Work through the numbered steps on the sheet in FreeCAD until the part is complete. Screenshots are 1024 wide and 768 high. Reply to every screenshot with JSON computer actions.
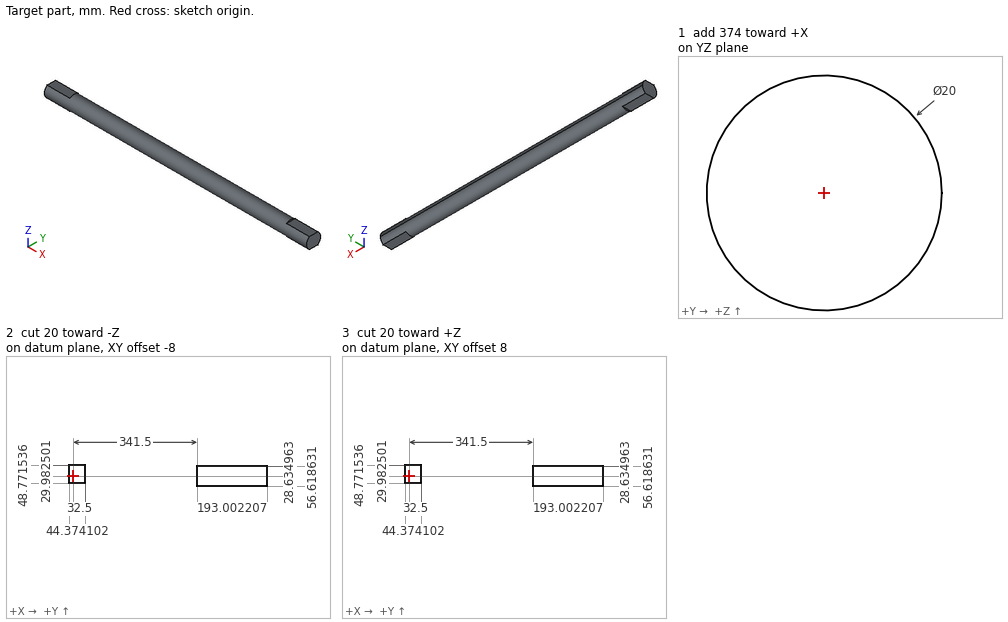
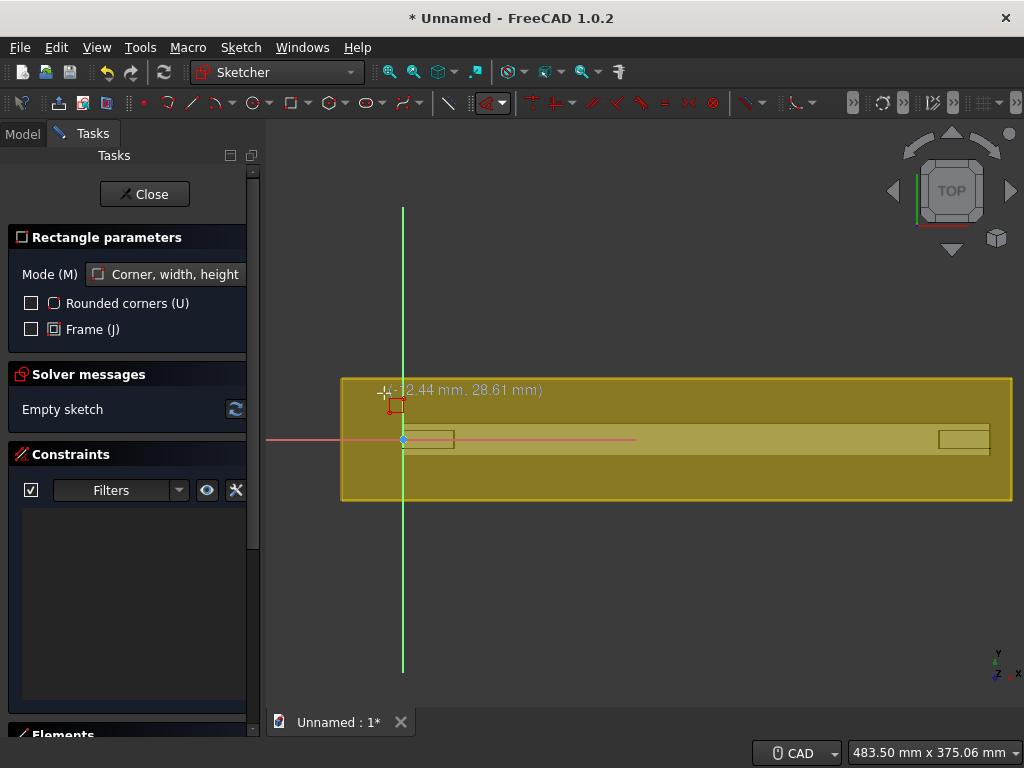
{"action": "left_click", "coordinate": [385, 393]}
{"action": "mouse_move", "coordinate": [454, 469]}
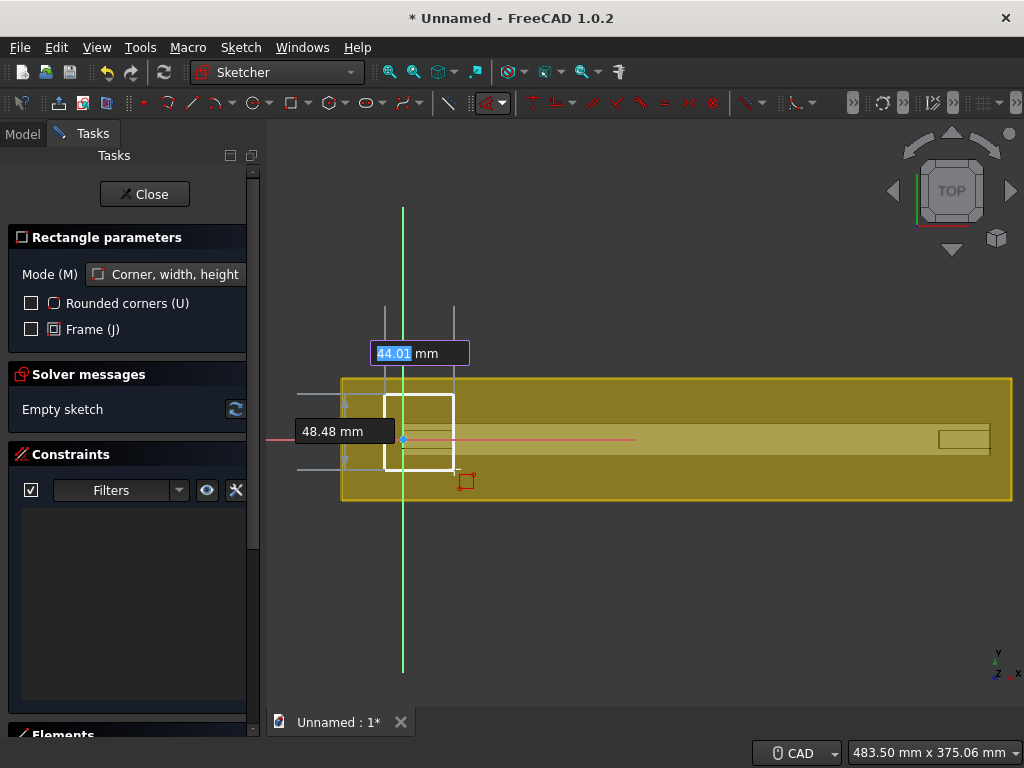
{"action": "type", "text": "44.374102"}
{"action": "key", "text": "Tab"}
{"action": "type", "text": "48.771536"}
{"action": "key", "text": "Return"}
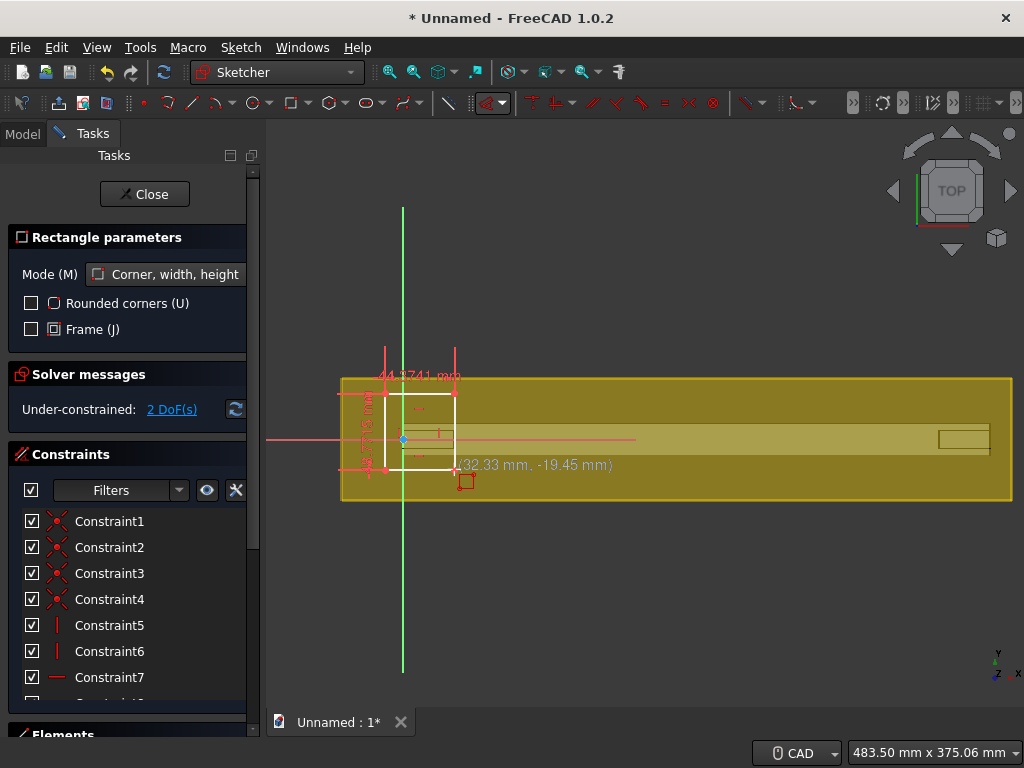
{"action": "scroll", "coordinate": [384, 393], "scroll_direction": "down", "scroll_amount": 4}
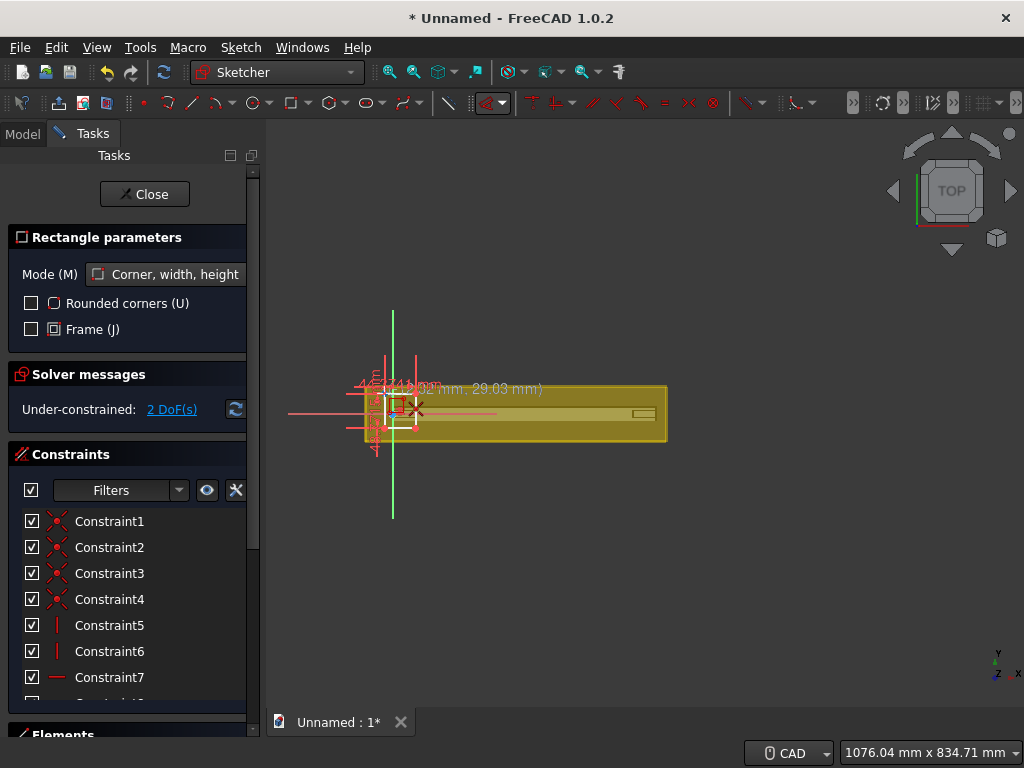
{"action": "left_click", "coordinate": [633, 394]}
{"action": "mouse_move", "coordinate": [769, 434]}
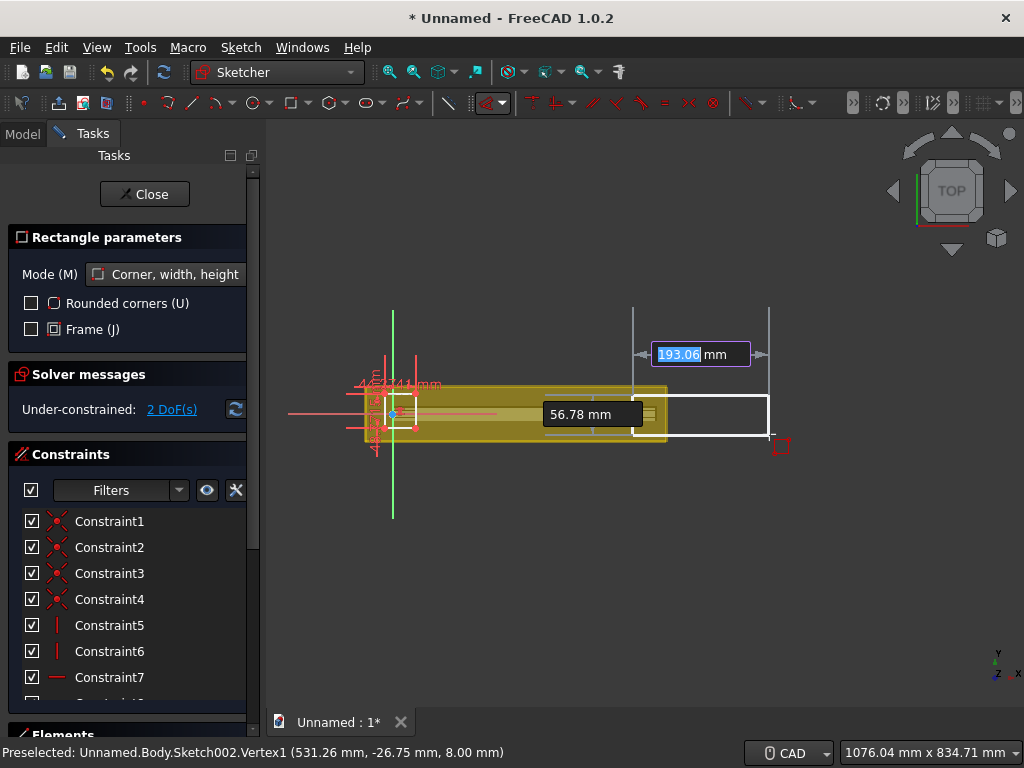
{"action": "type", "text": "193.002207"}
{"action": "key", "text": "Tab"}
{"action": "type", "text": "56.618631"}
{"action": "key", "text": "Return"}
{"action": "key", "text": "Escape"}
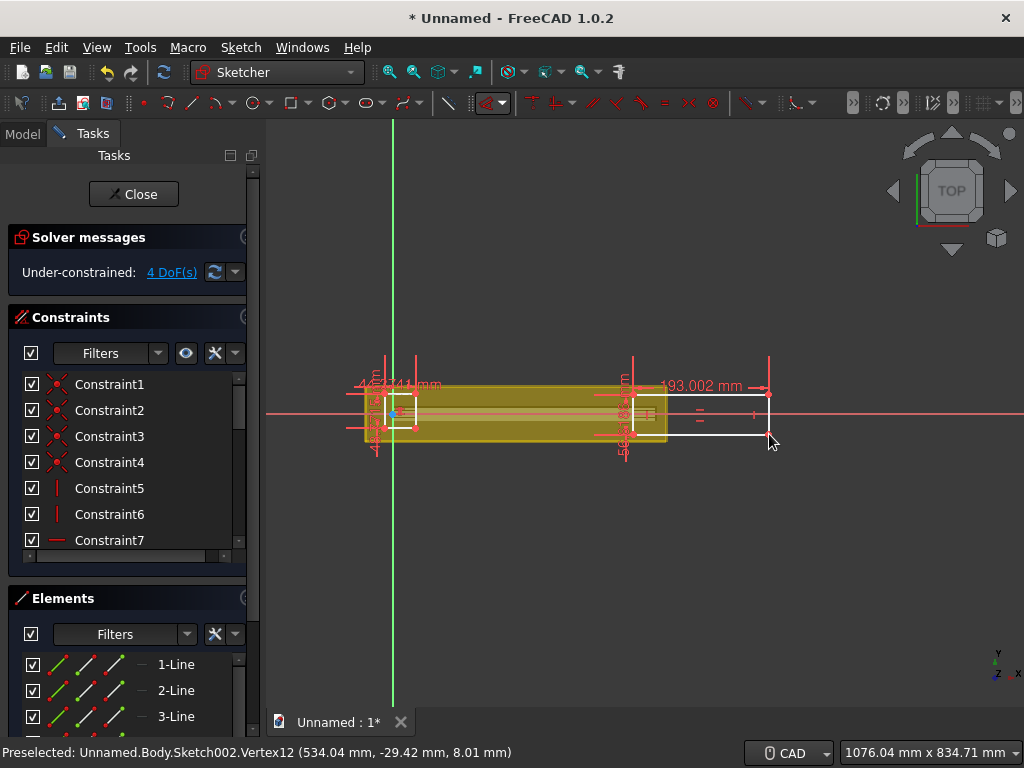
{"action": "scroll", "coordinate": [416, 428], "scroll_direction": "up", "scroll_amount": 3}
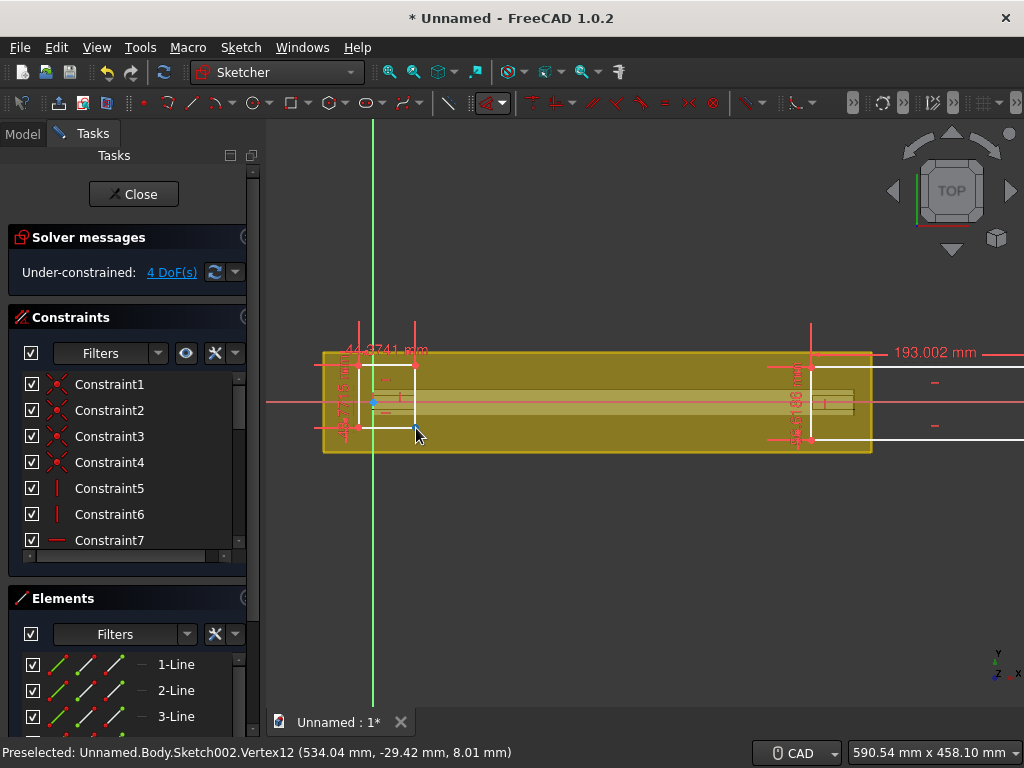
{"action": "left_click", "coordinate": [415, 428]}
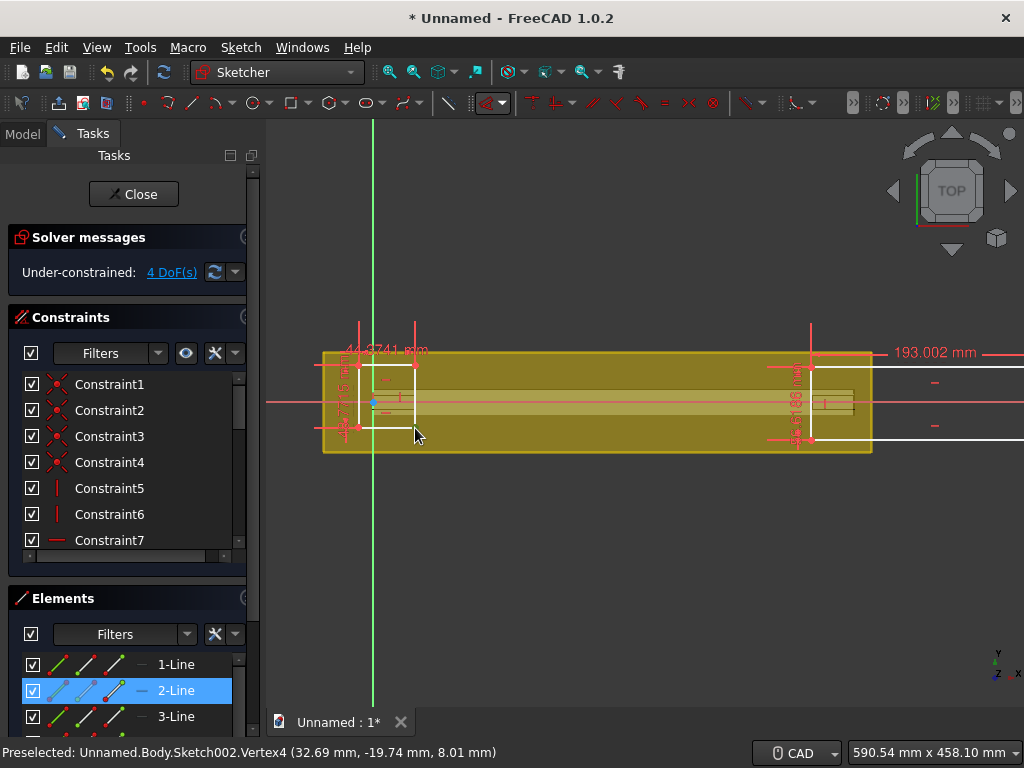
{"action": "left_click", "coordinate": [504, 104]}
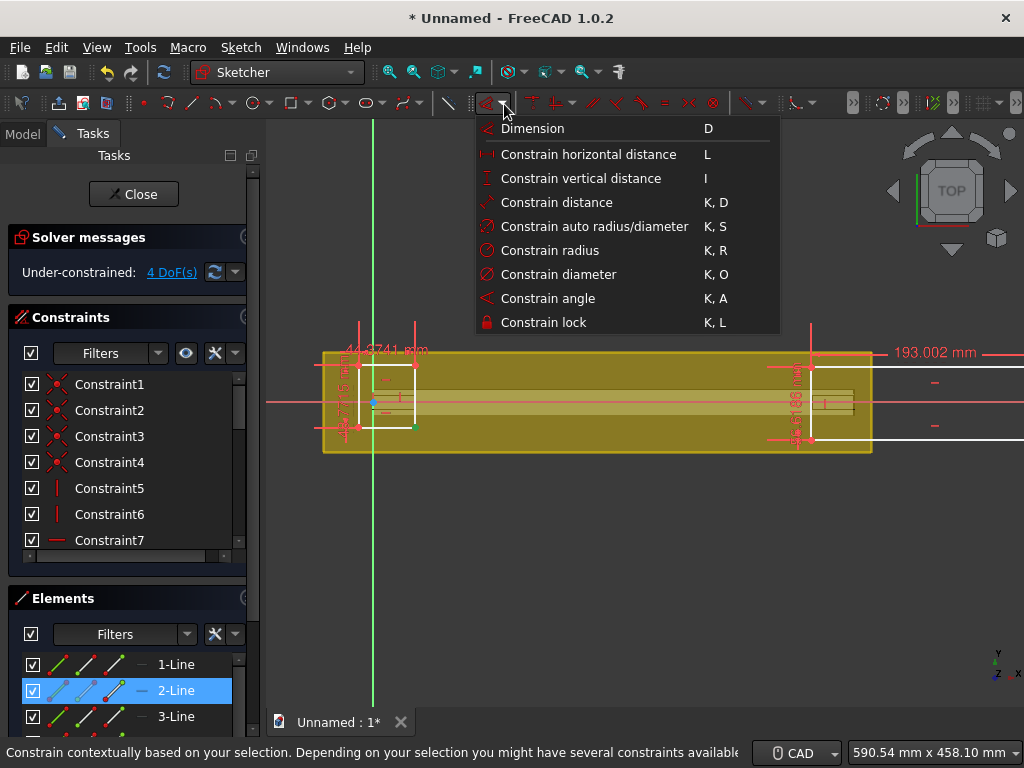
{"action": "left_click", "coordinate": [628, 154]}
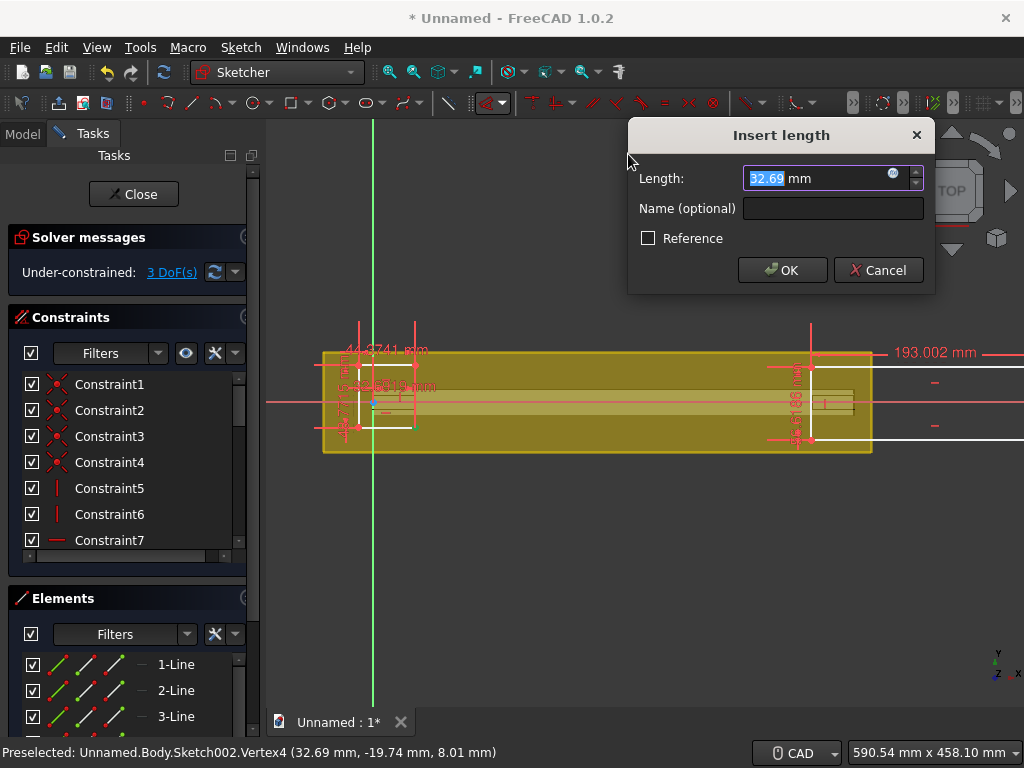
{"action": "type", "text": "32.5"}
{"action": "key", "text": "Return"}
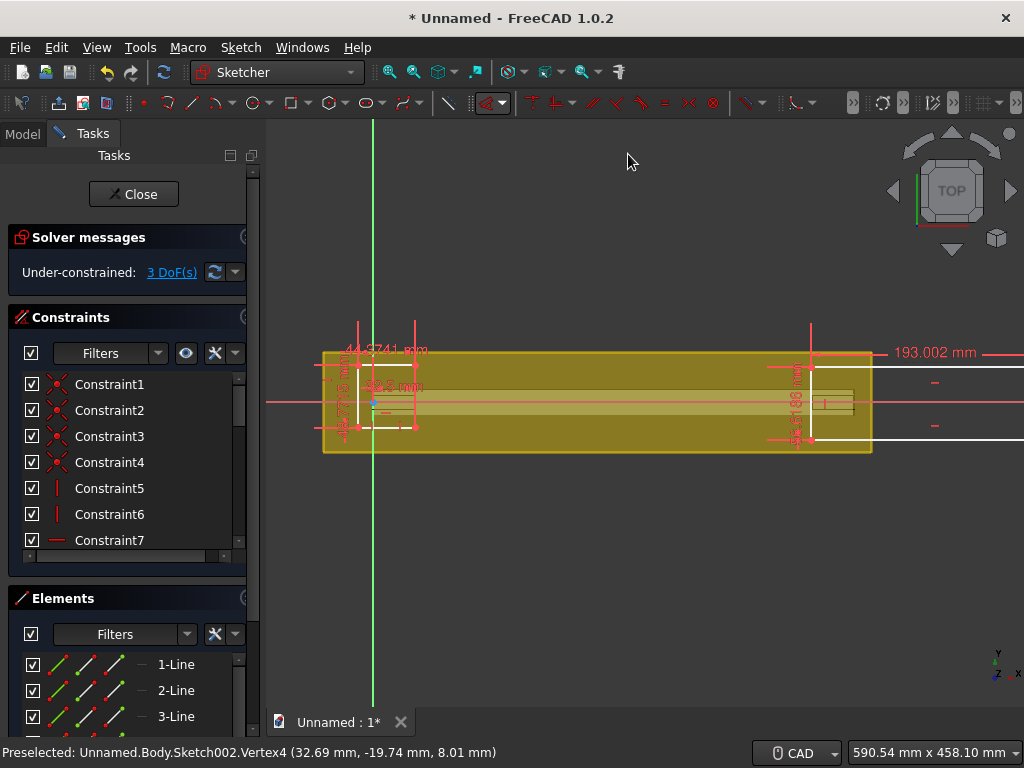
{"action": "left_click", "coordinate": [811, 367]}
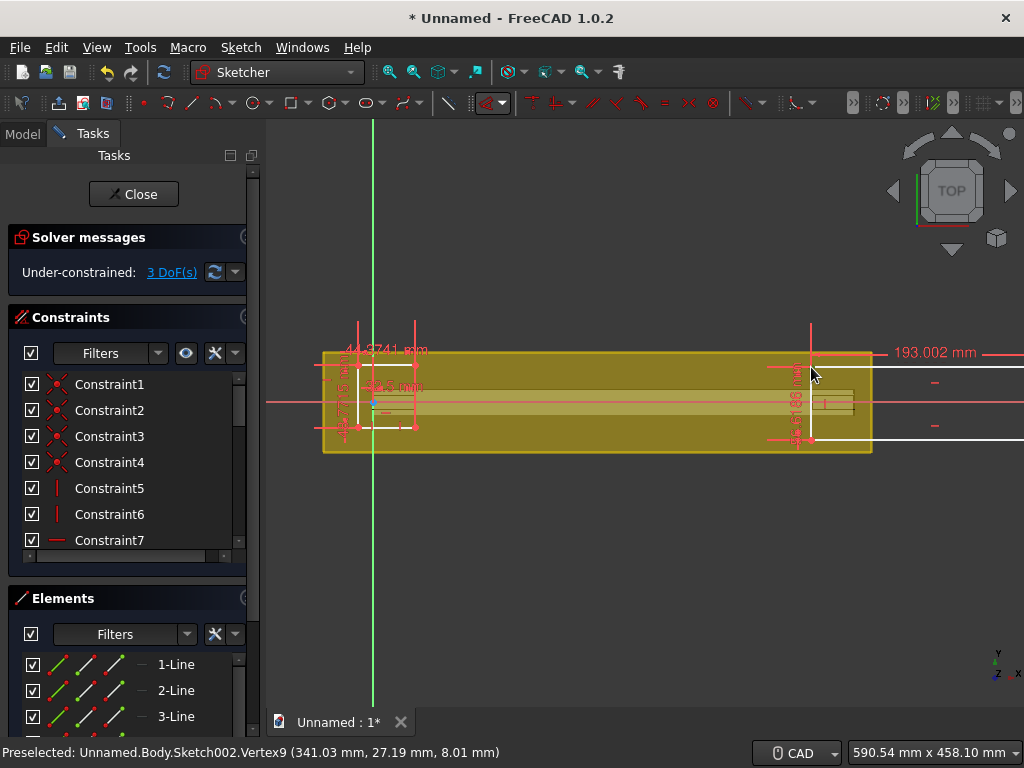
{"action": "key", "text": "l"}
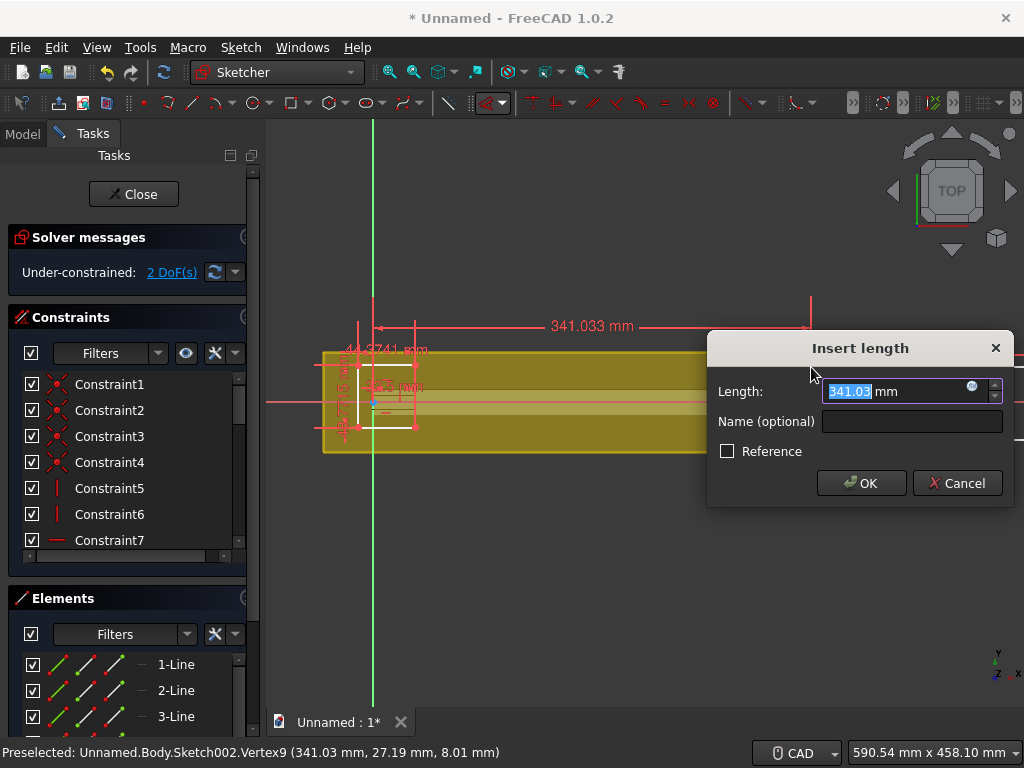
{"action": "type", "text": "341.5"}
{"action": "key", "text": "Return"}